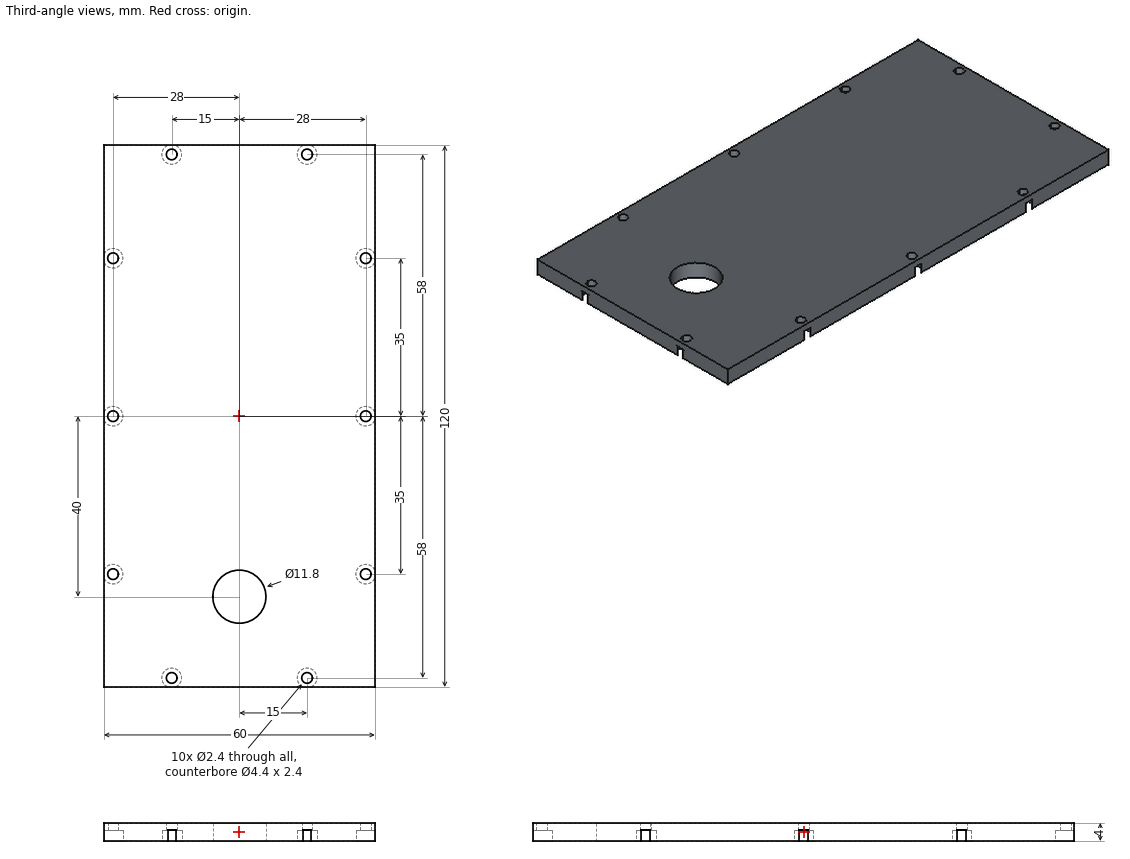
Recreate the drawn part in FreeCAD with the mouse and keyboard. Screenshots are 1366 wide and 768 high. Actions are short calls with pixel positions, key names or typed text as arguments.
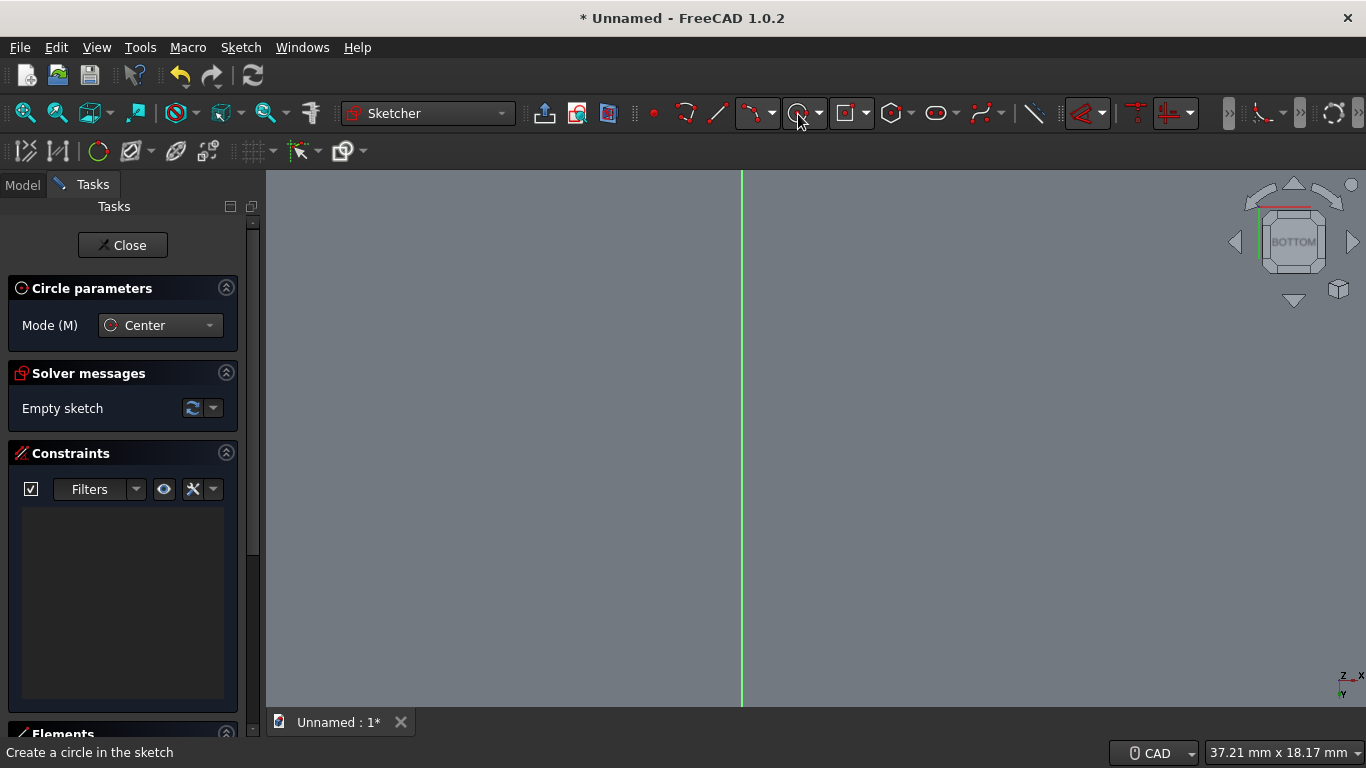
click(742, 440)
click(866, 317)
key(Escape)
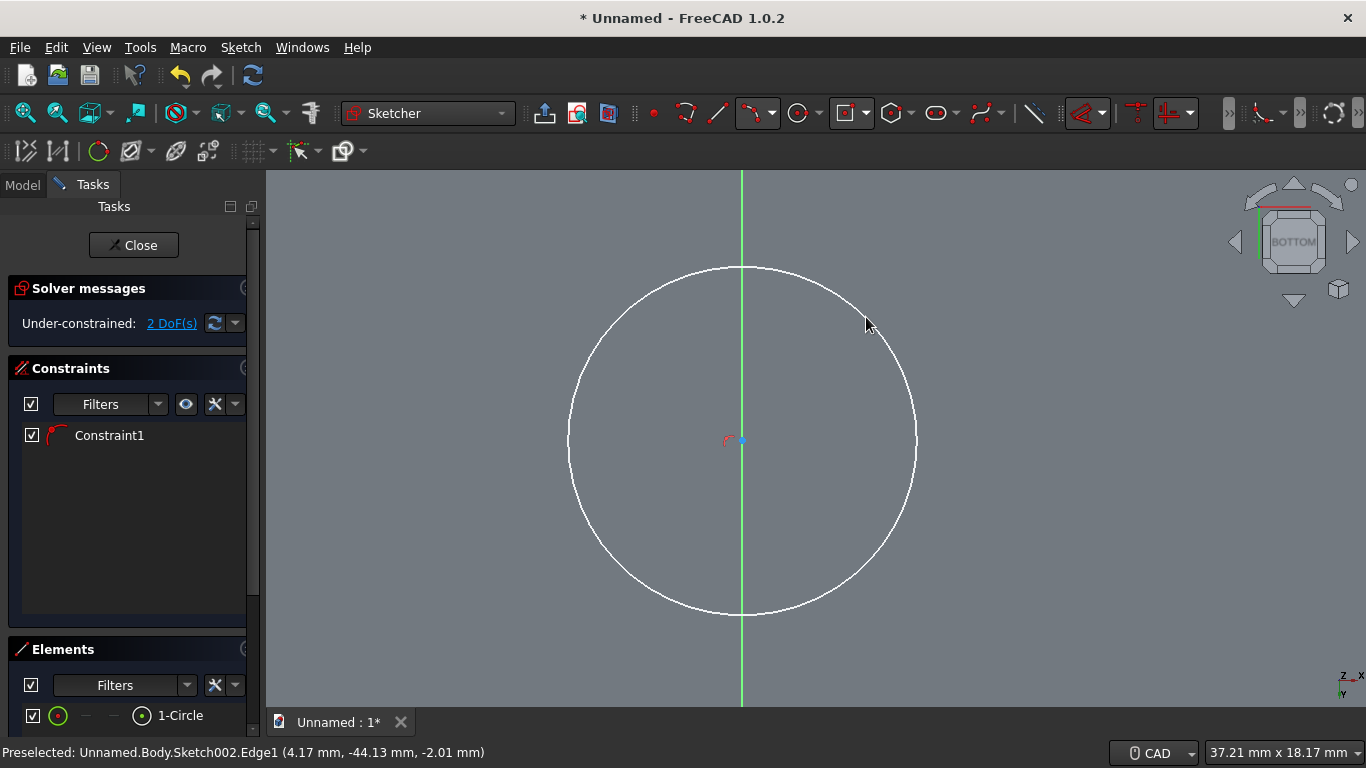
click(865, 317)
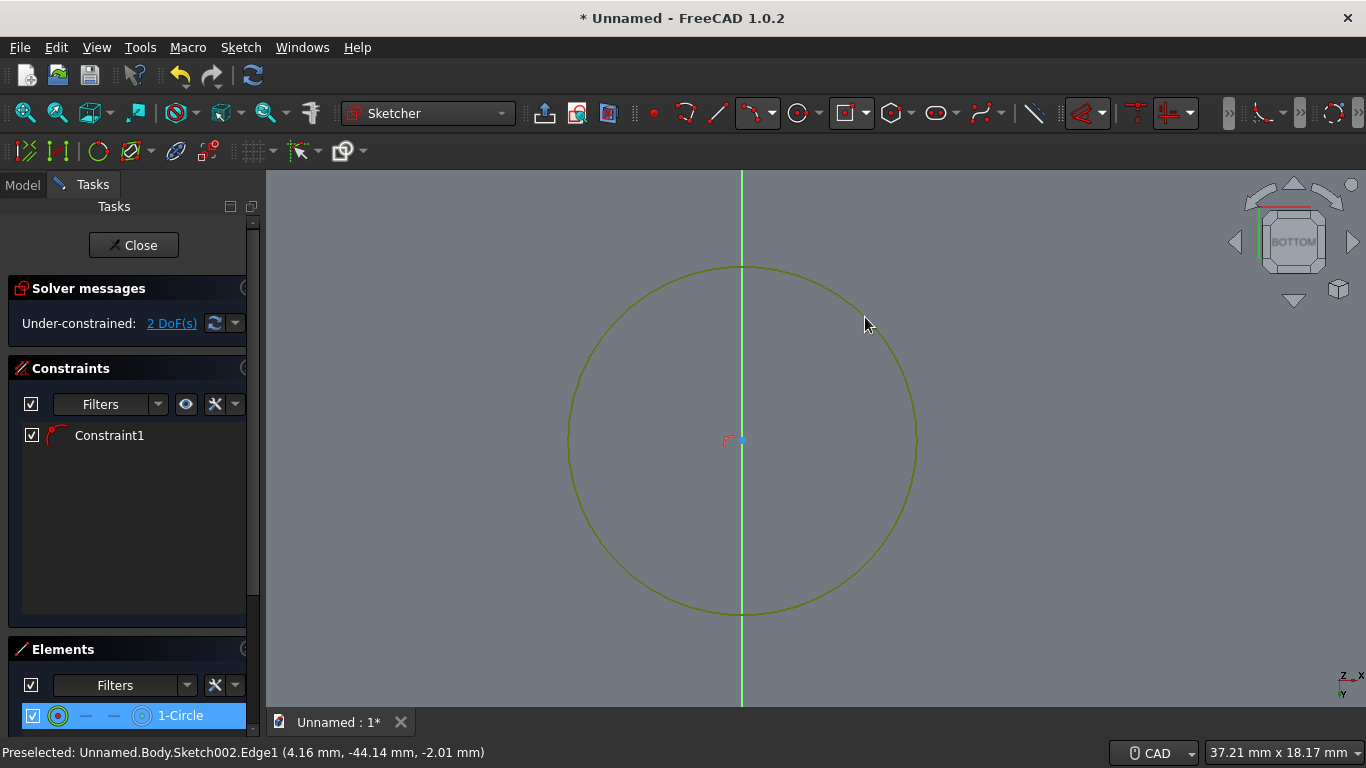
click(1104, 114)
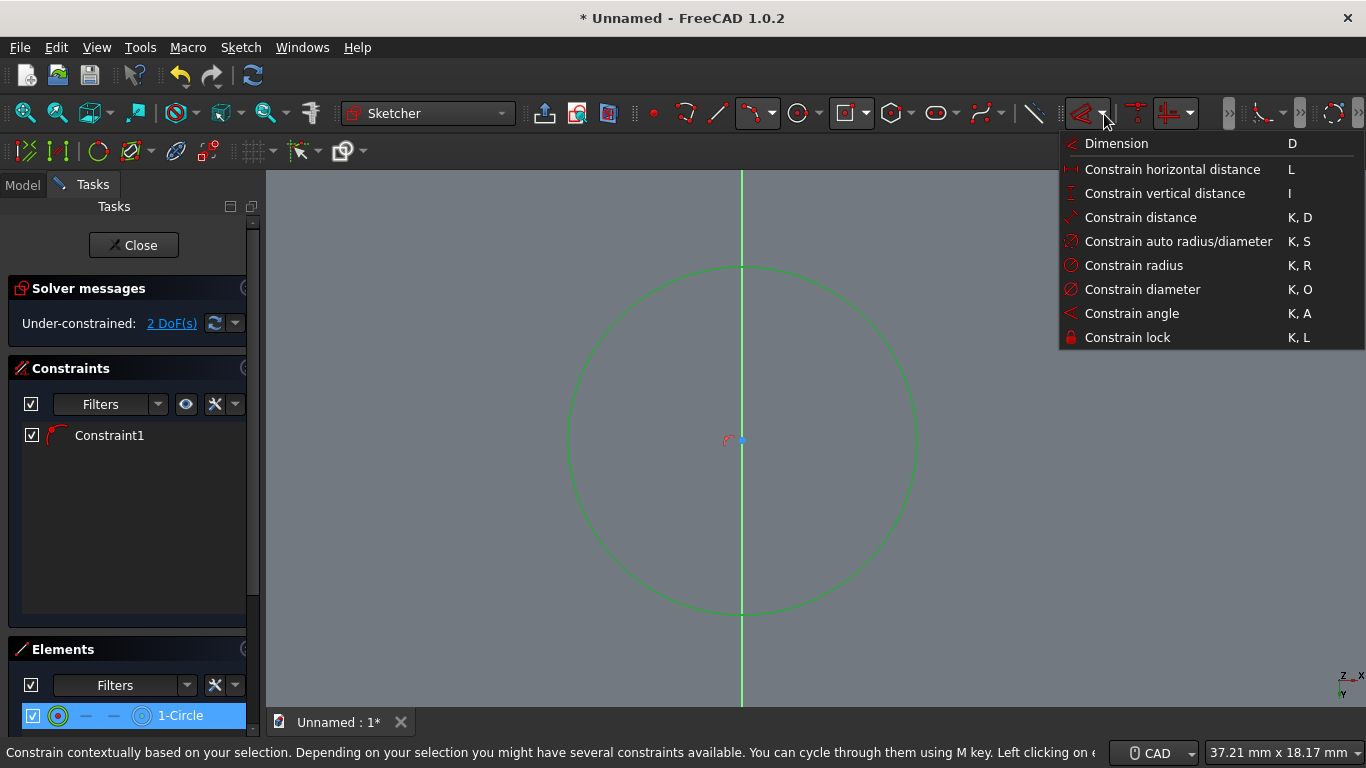
click(1212, 289)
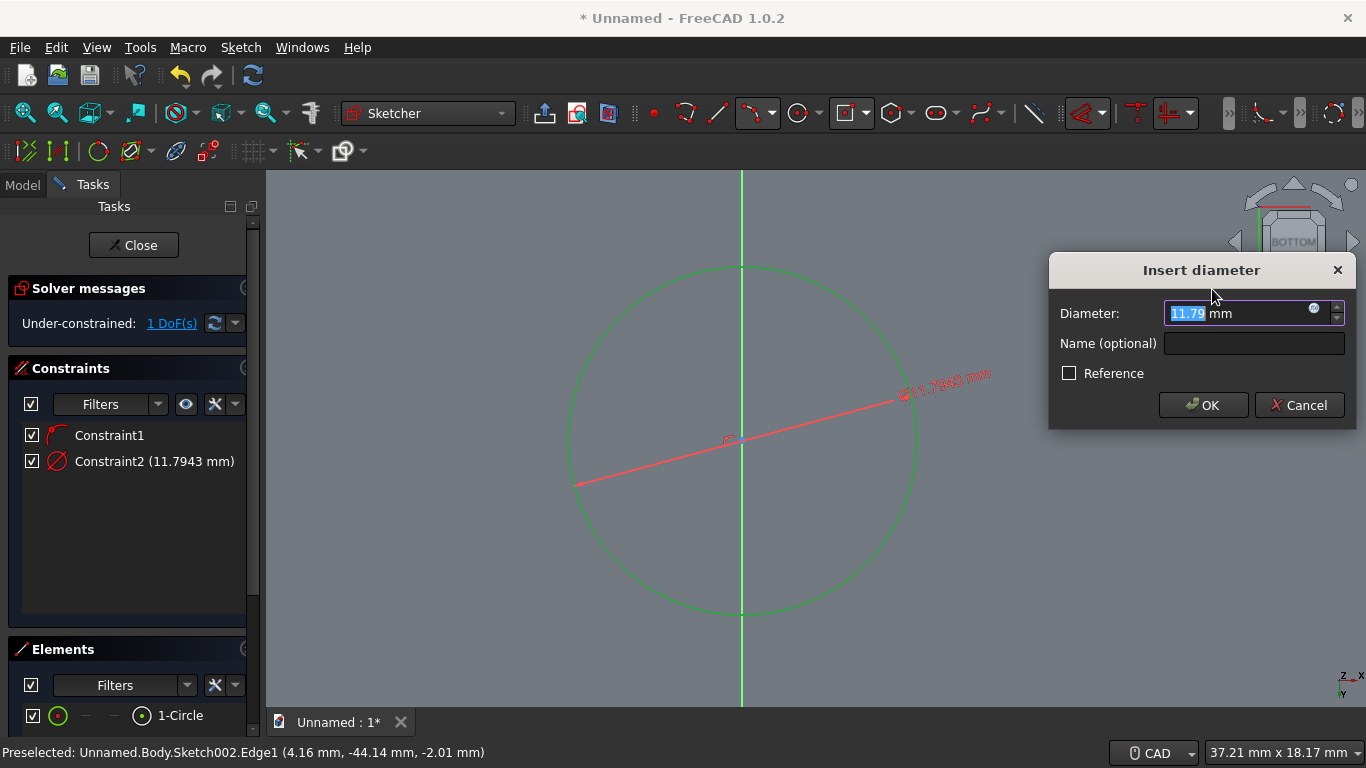
text(11.8)
key(Return)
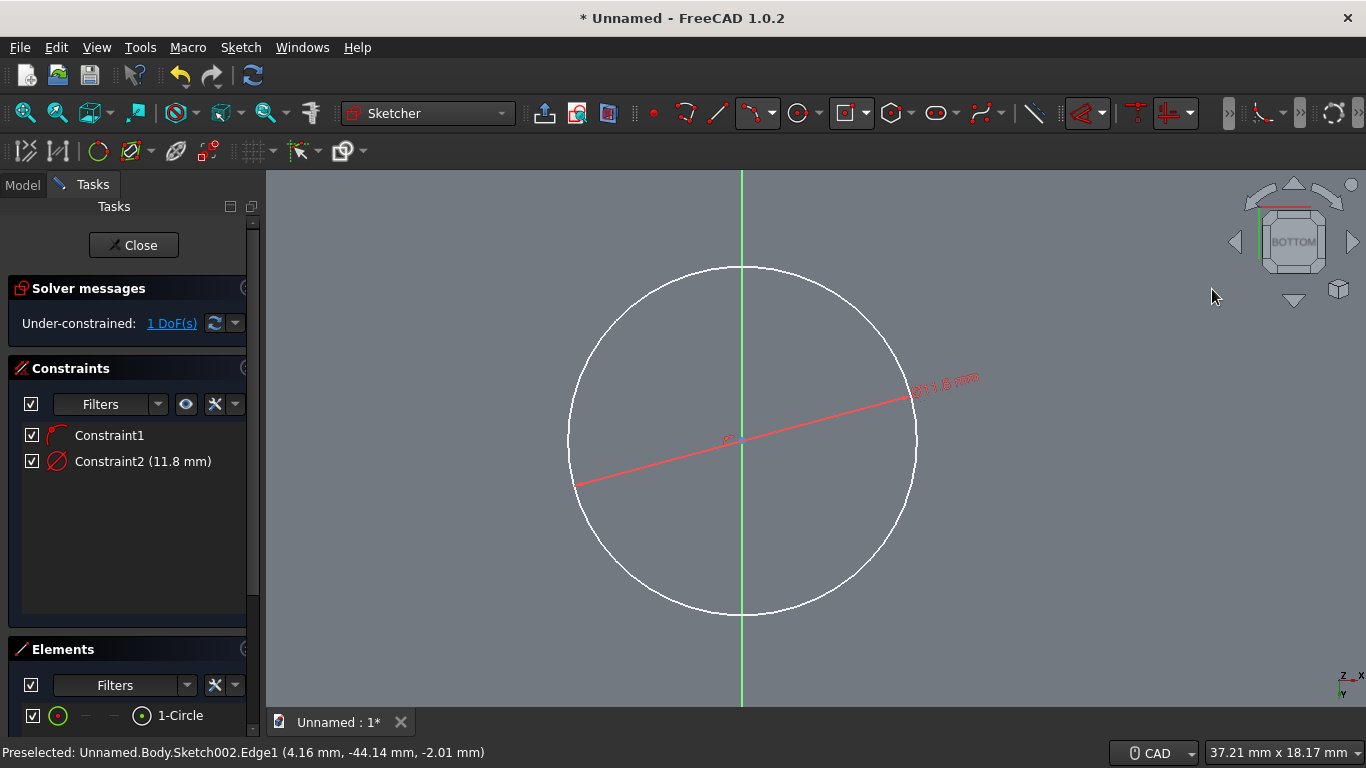
click(742, 441)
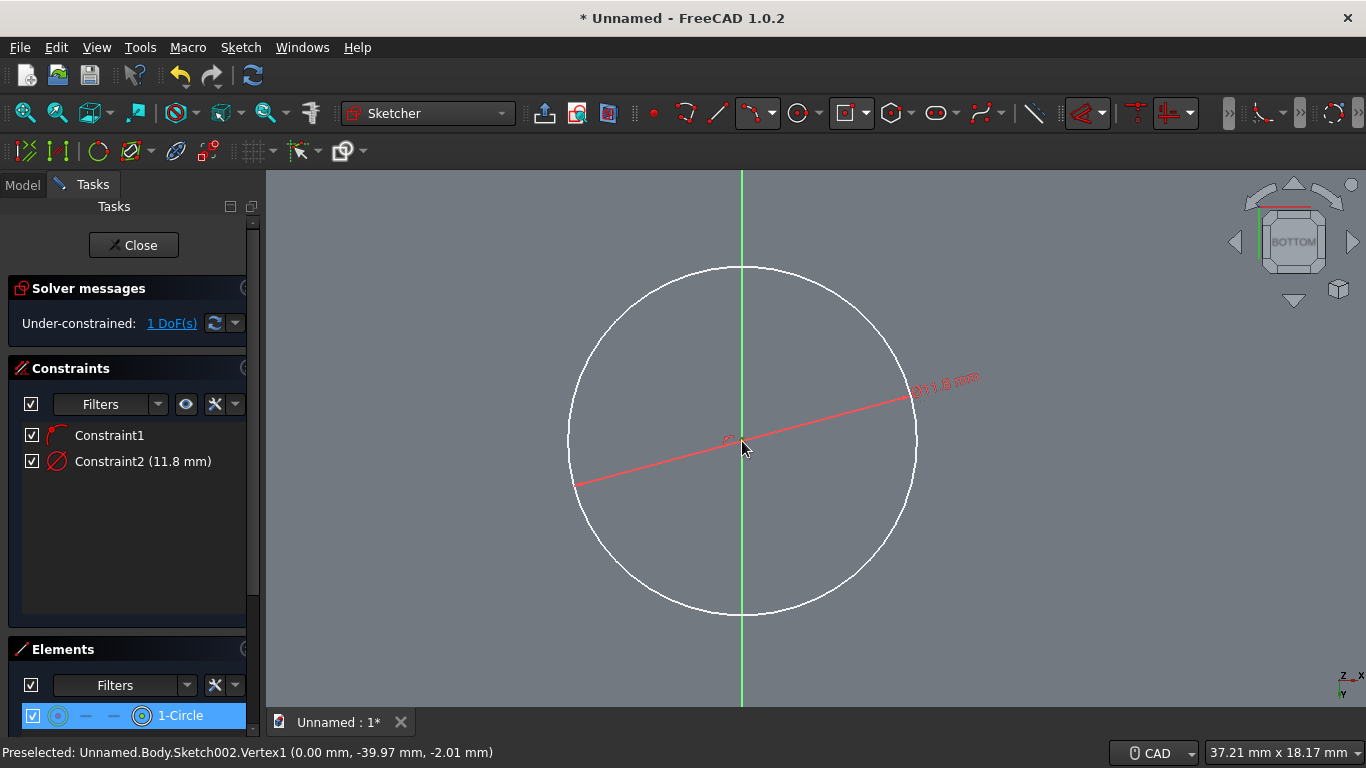
key(i)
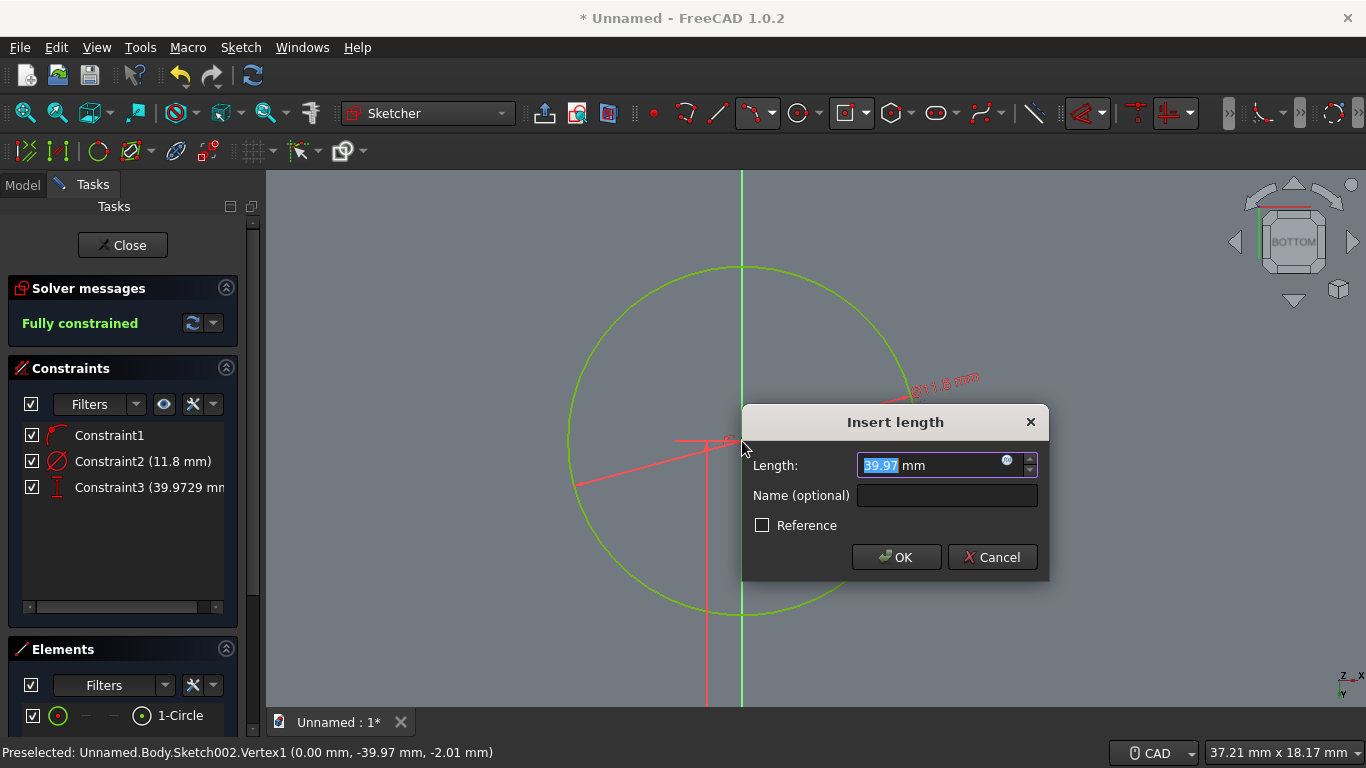
text(40)
key(Return)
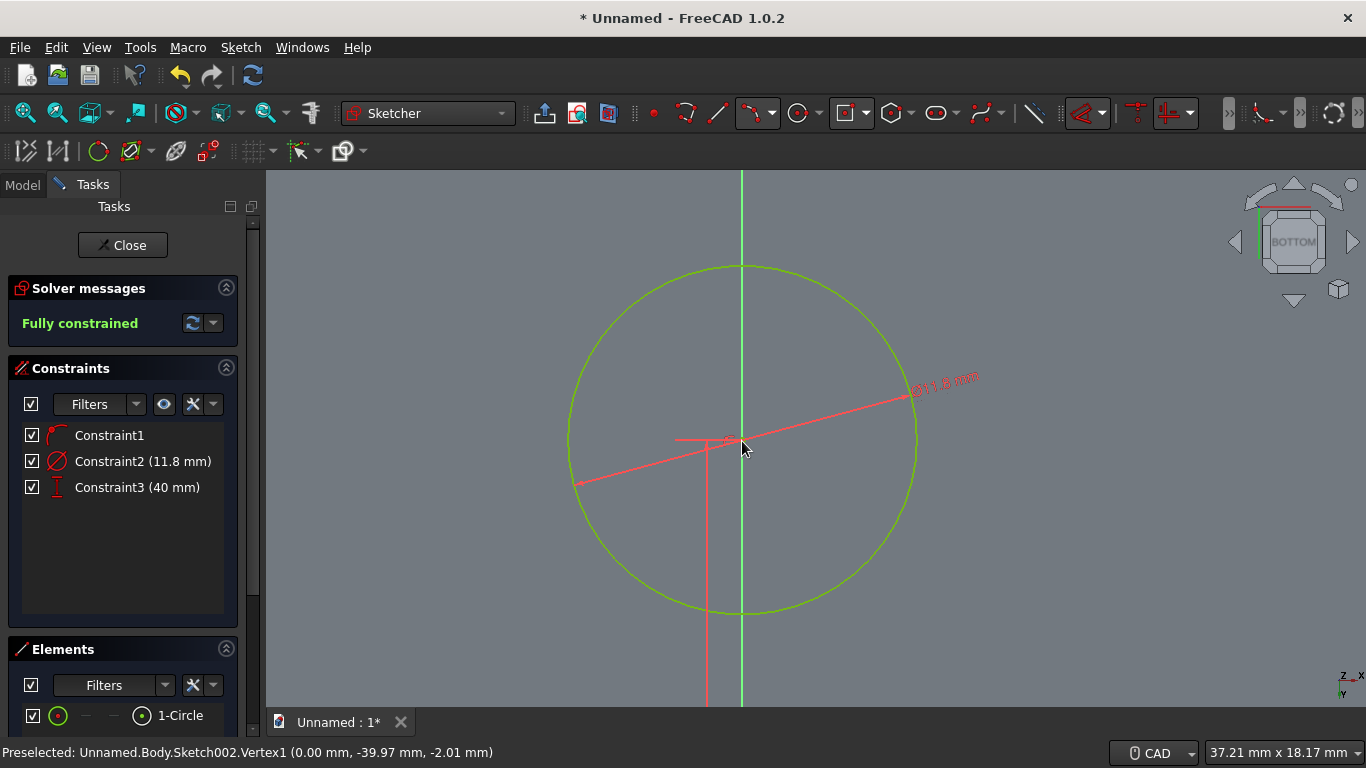
click(123, 245)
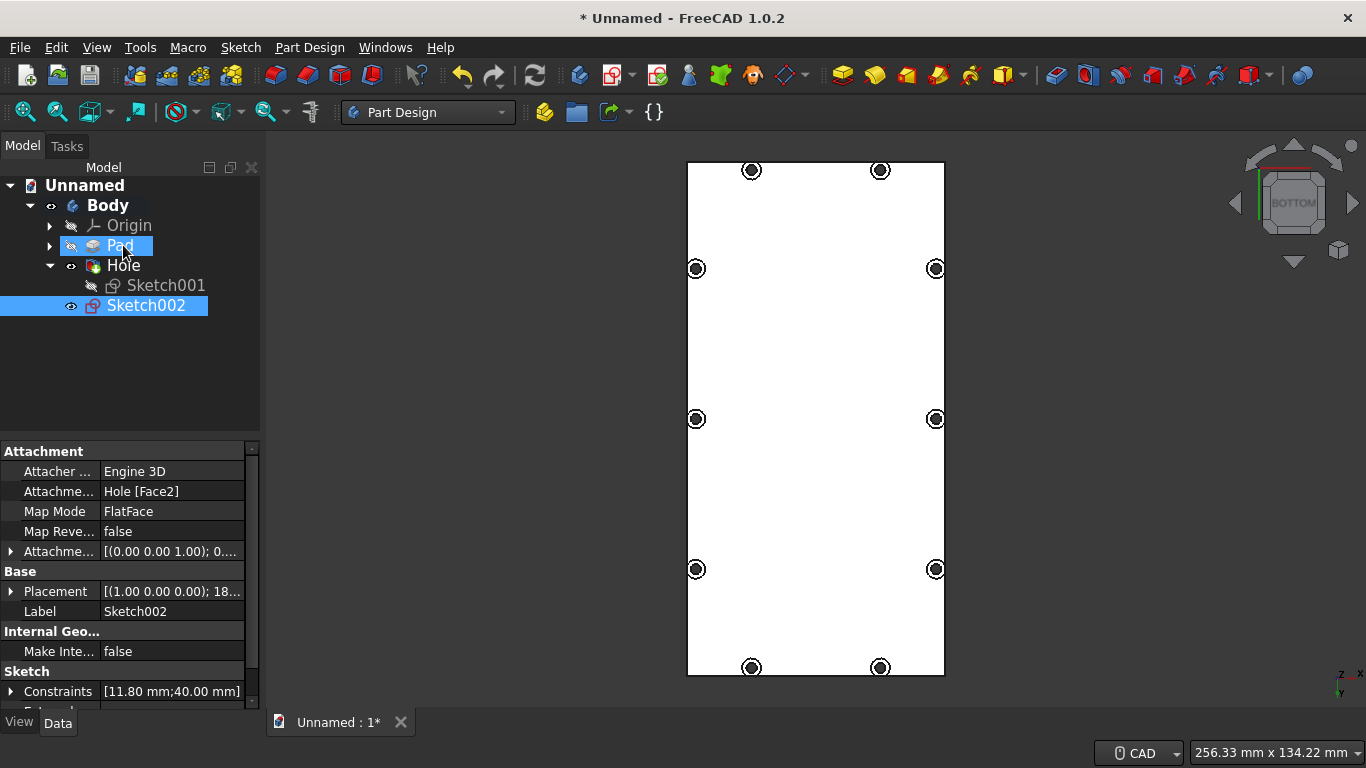
click(1058, 76)